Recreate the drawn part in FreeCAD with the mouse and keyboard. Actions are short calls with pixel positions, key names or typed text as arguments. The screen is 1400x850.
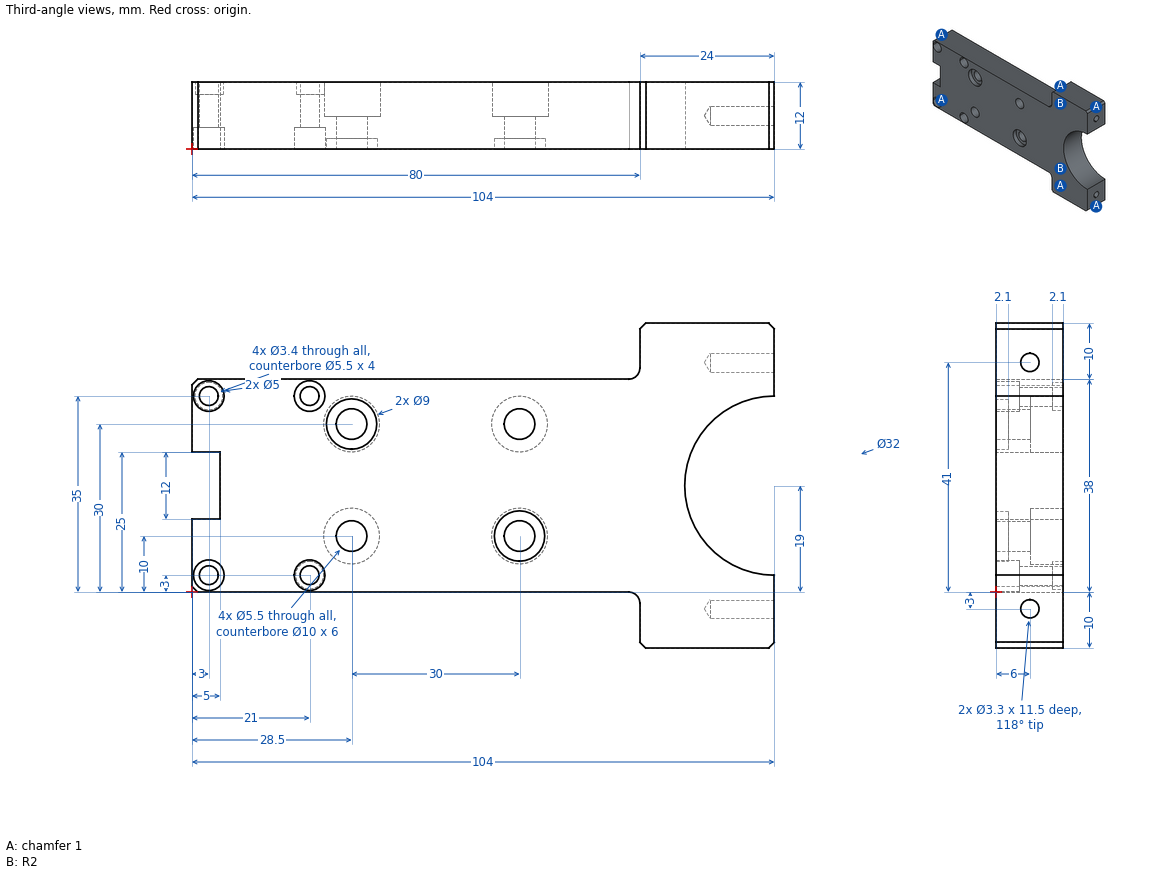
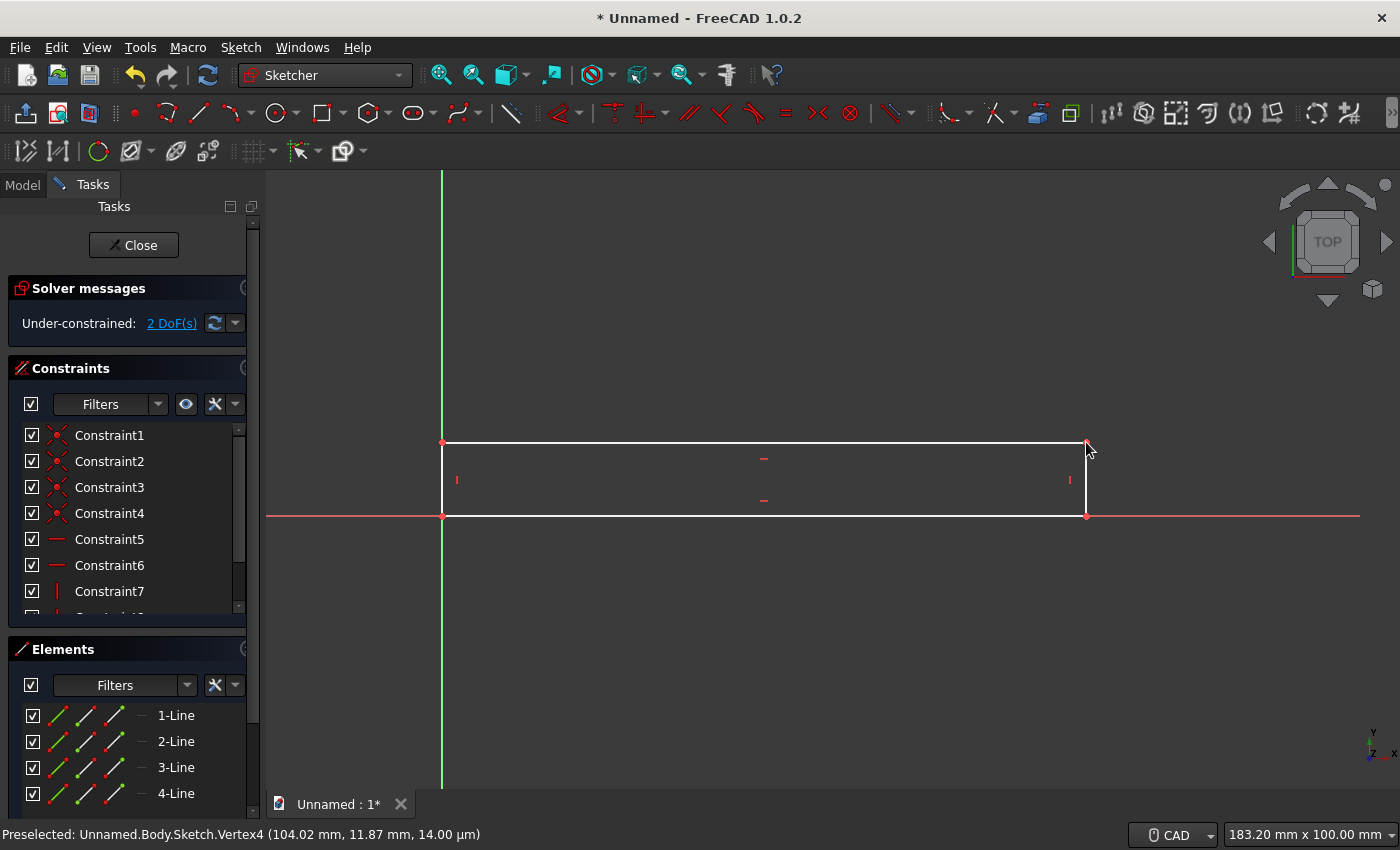
click(1086, 494)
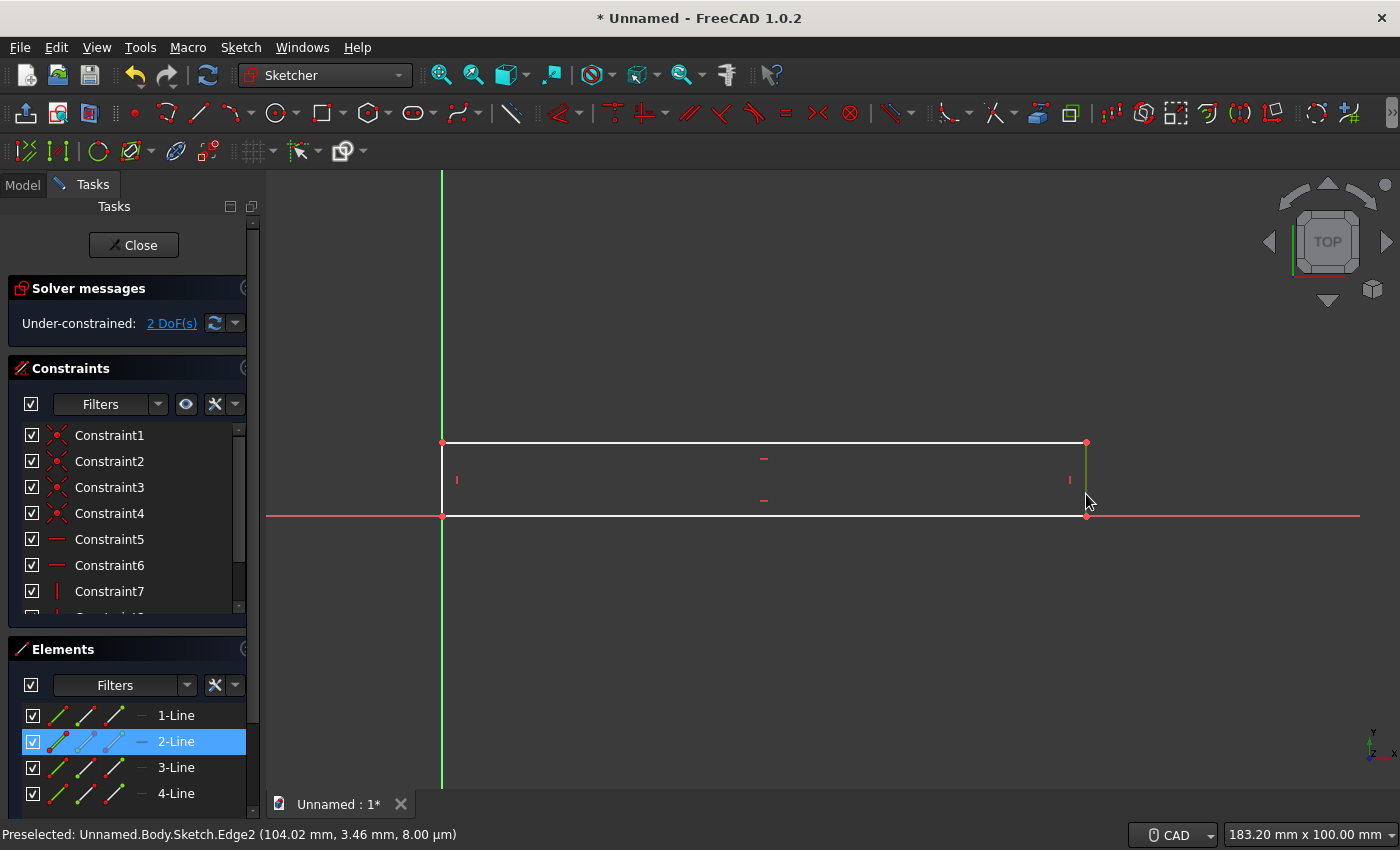
click(582, 114)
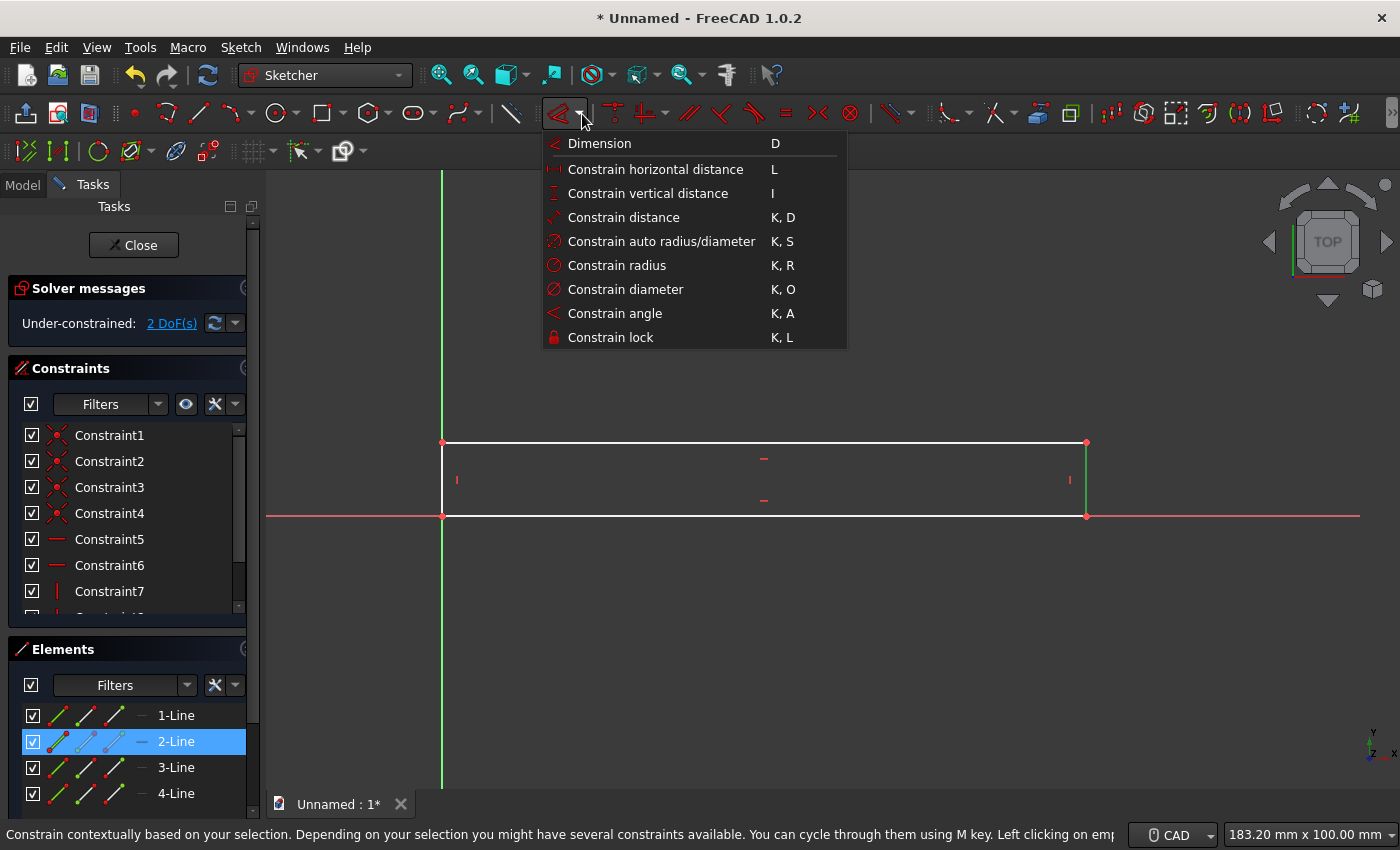
click(695, 193)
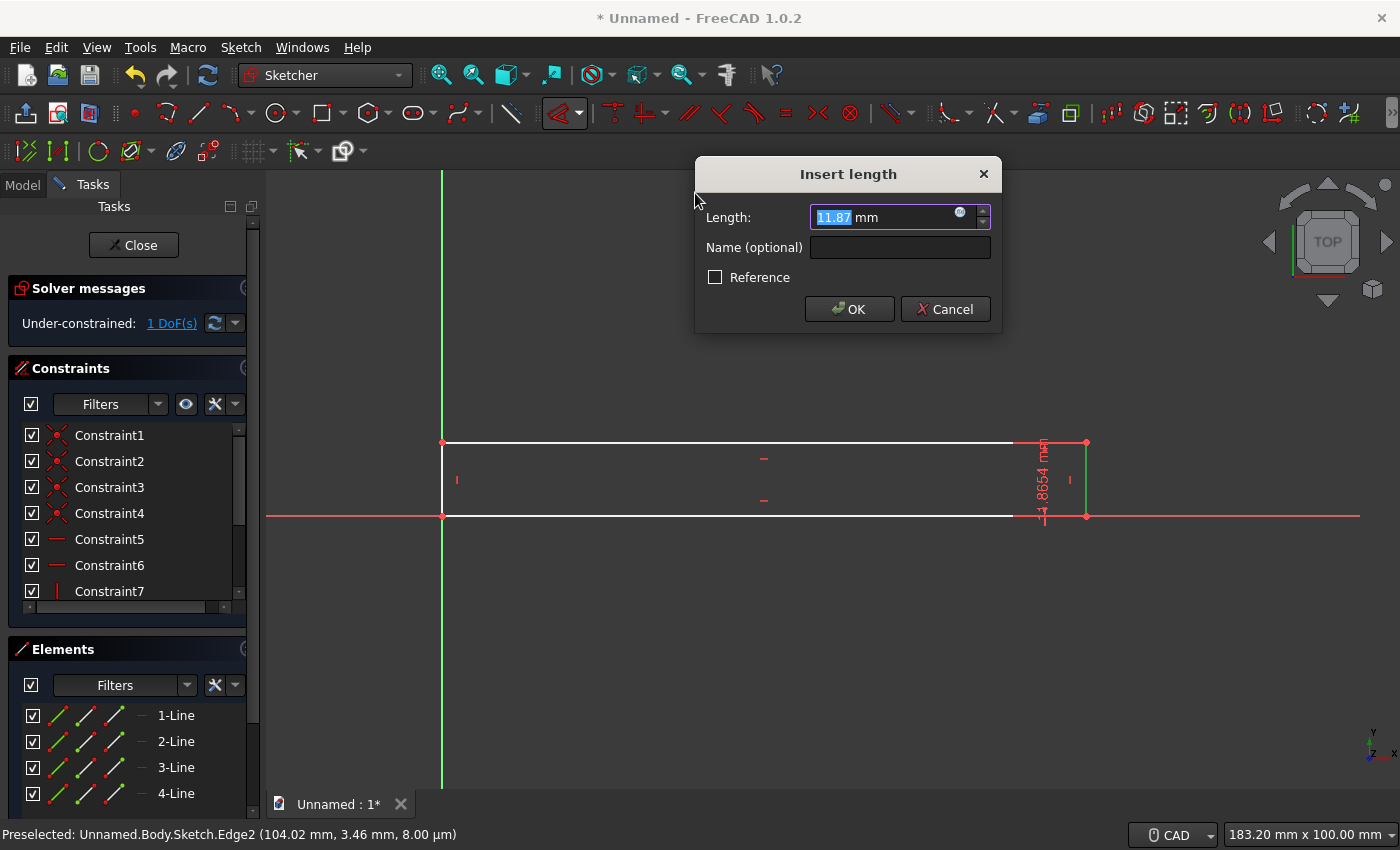
text(12)
key(Return)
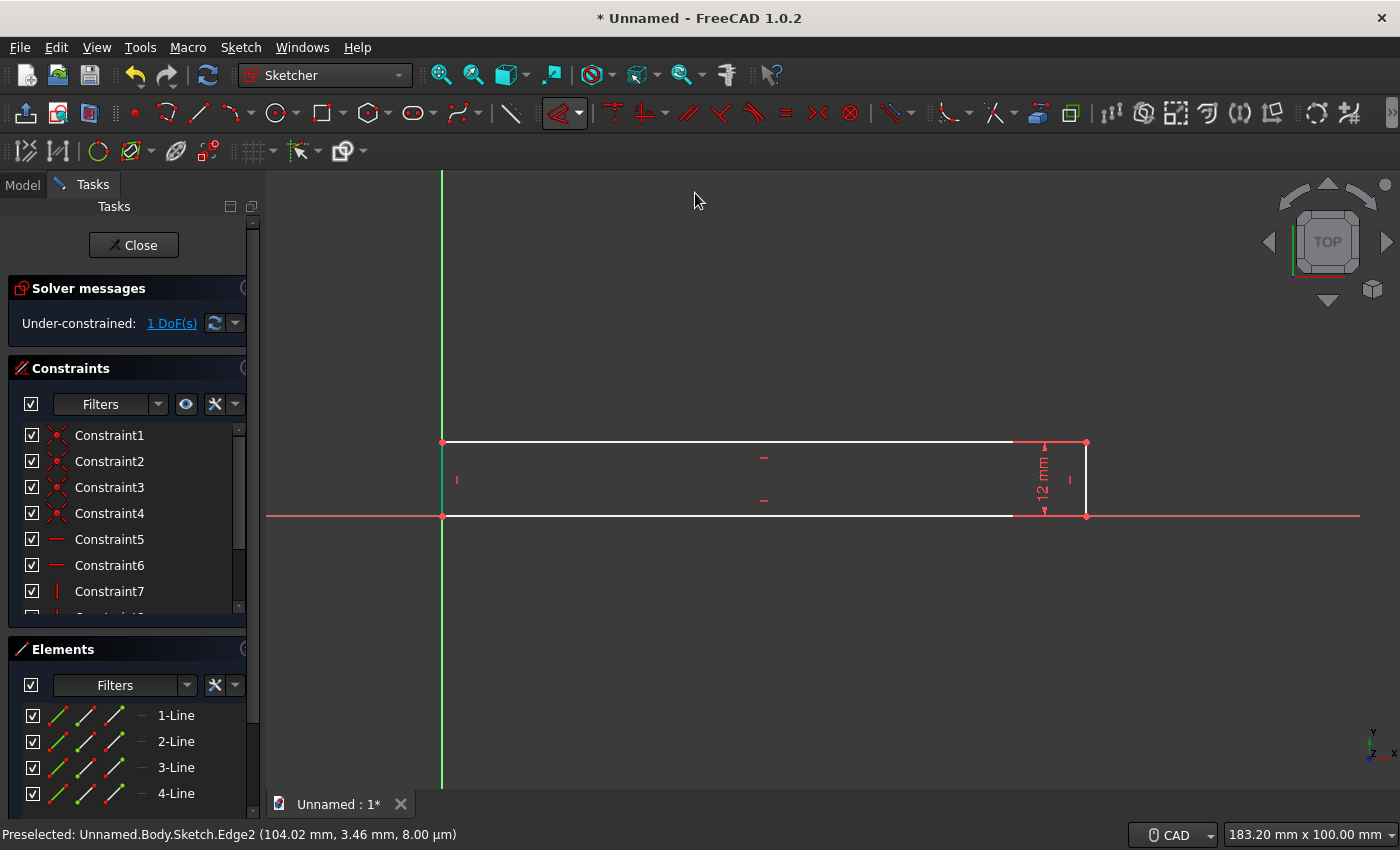
click(635, 516)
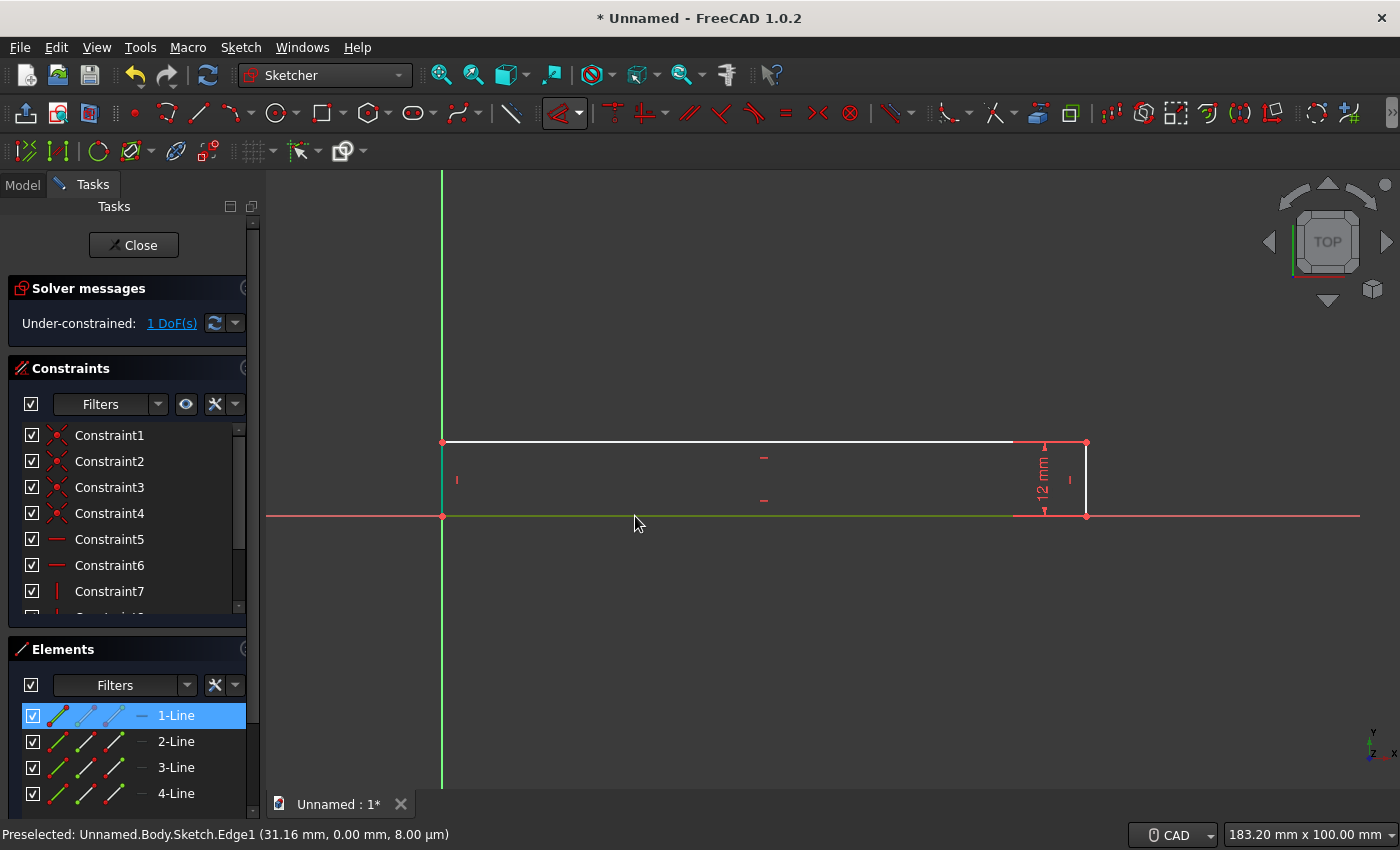
click(582, 114)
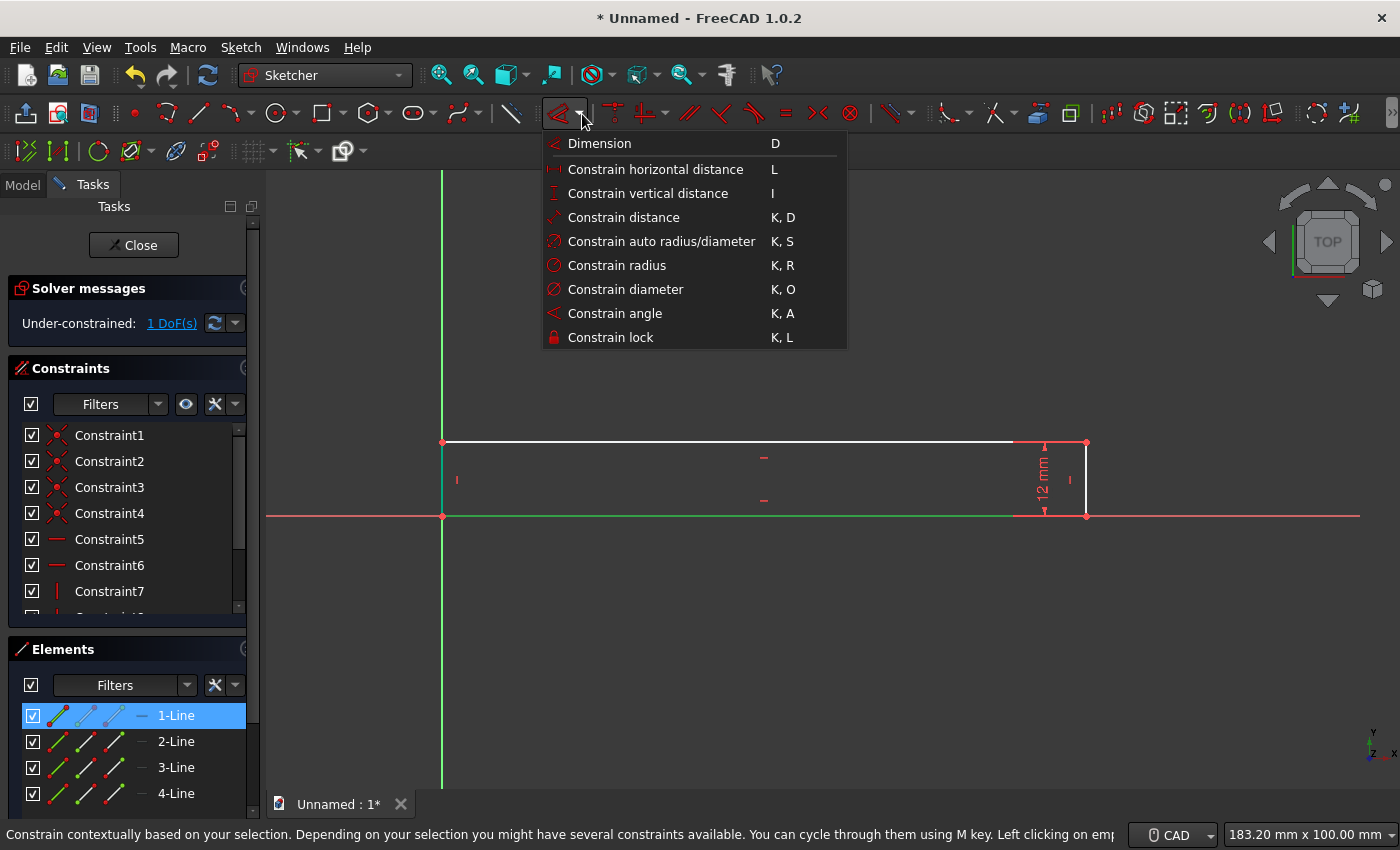
click(695, 169)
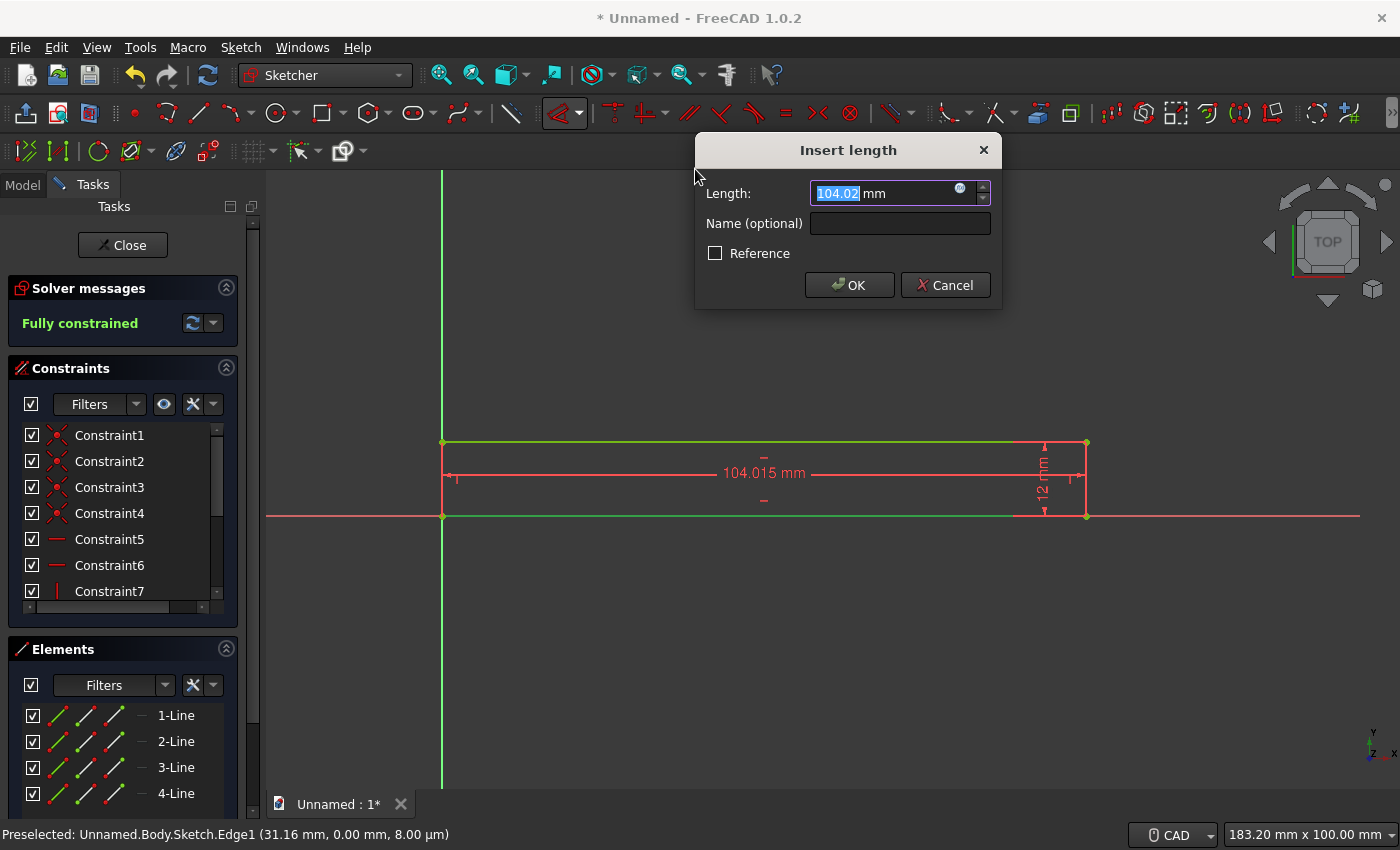
text(104)
key(Return)